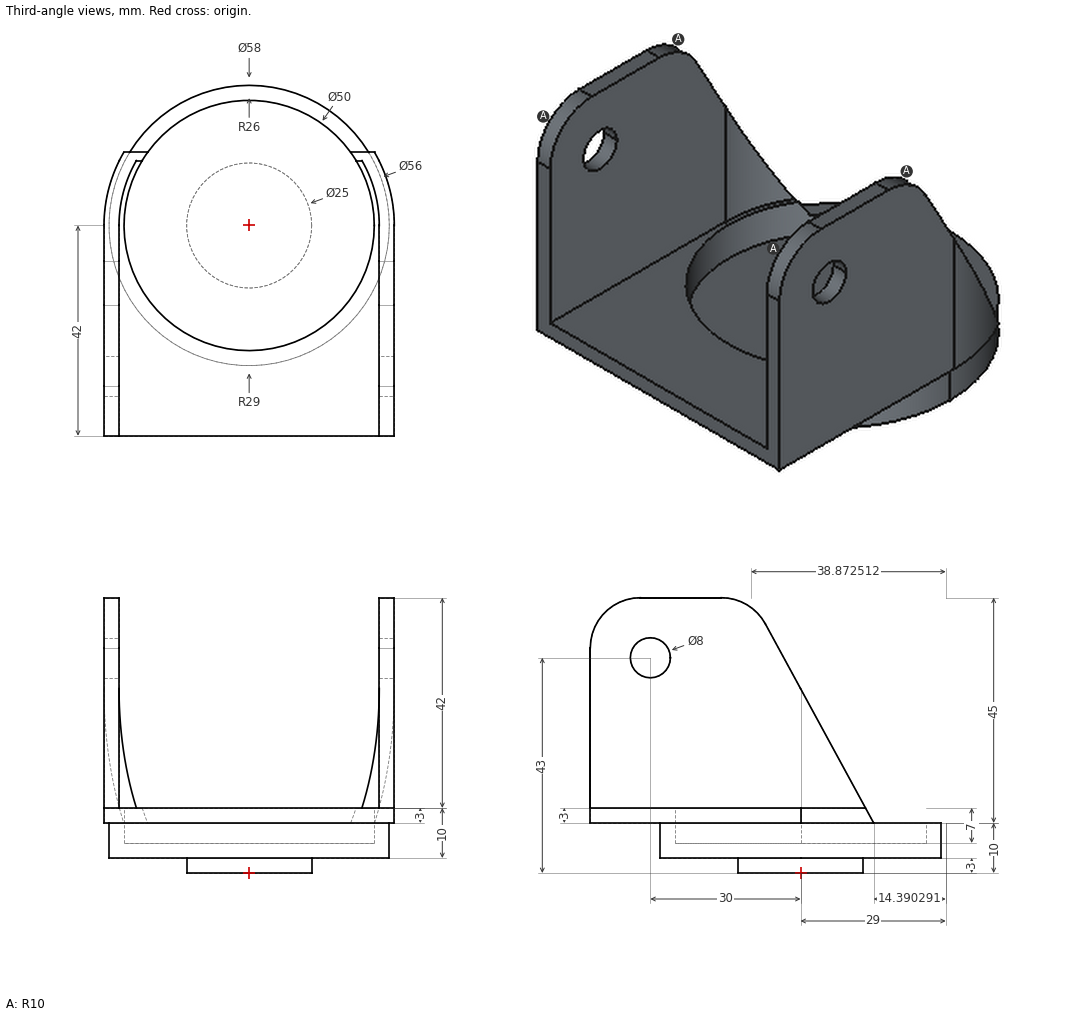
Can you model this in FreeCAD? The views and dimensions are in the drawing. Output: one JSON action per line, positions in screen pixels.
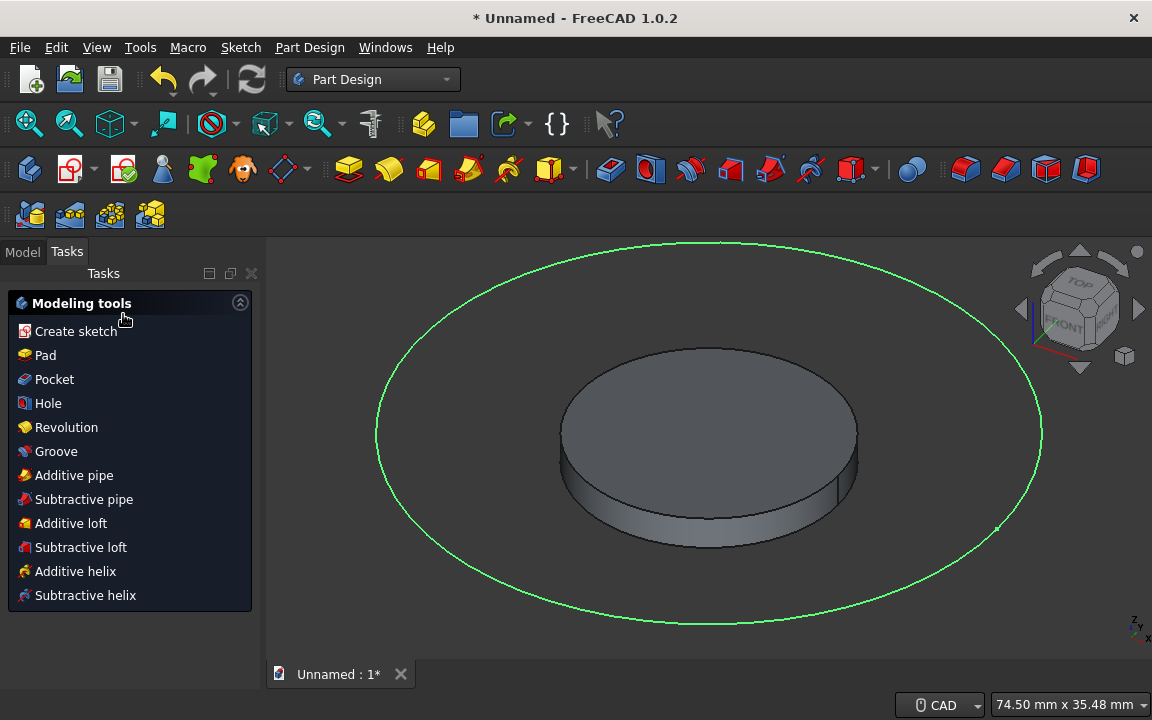
{"action": "left_click", "coordinate": [350, 170]}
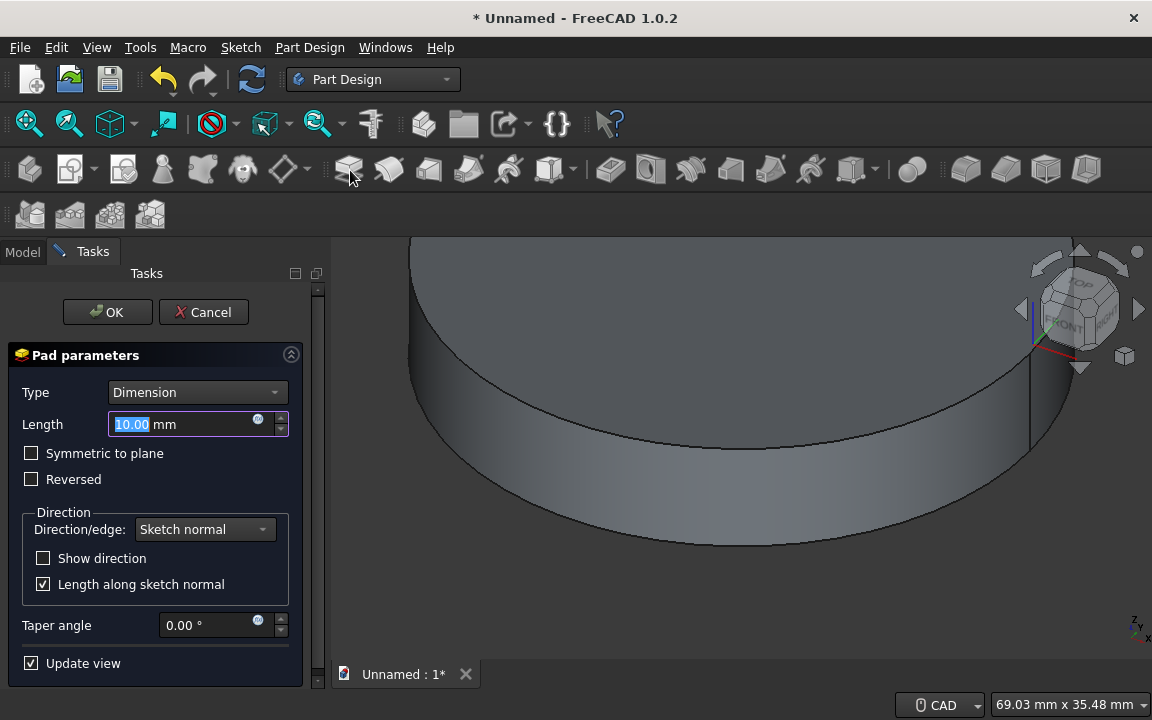
{"action": "type", "text": "10"}
{"action": "key", "text": "Tab"}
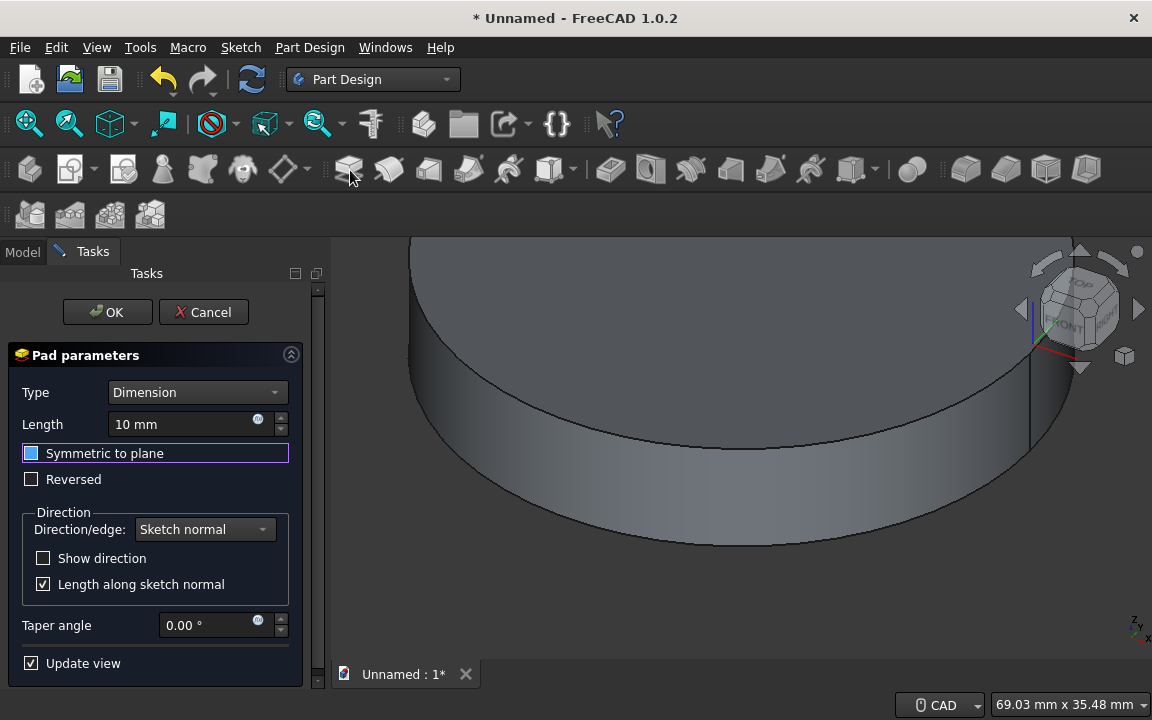
{"action": "left_click", "coordinate": [108, 312]}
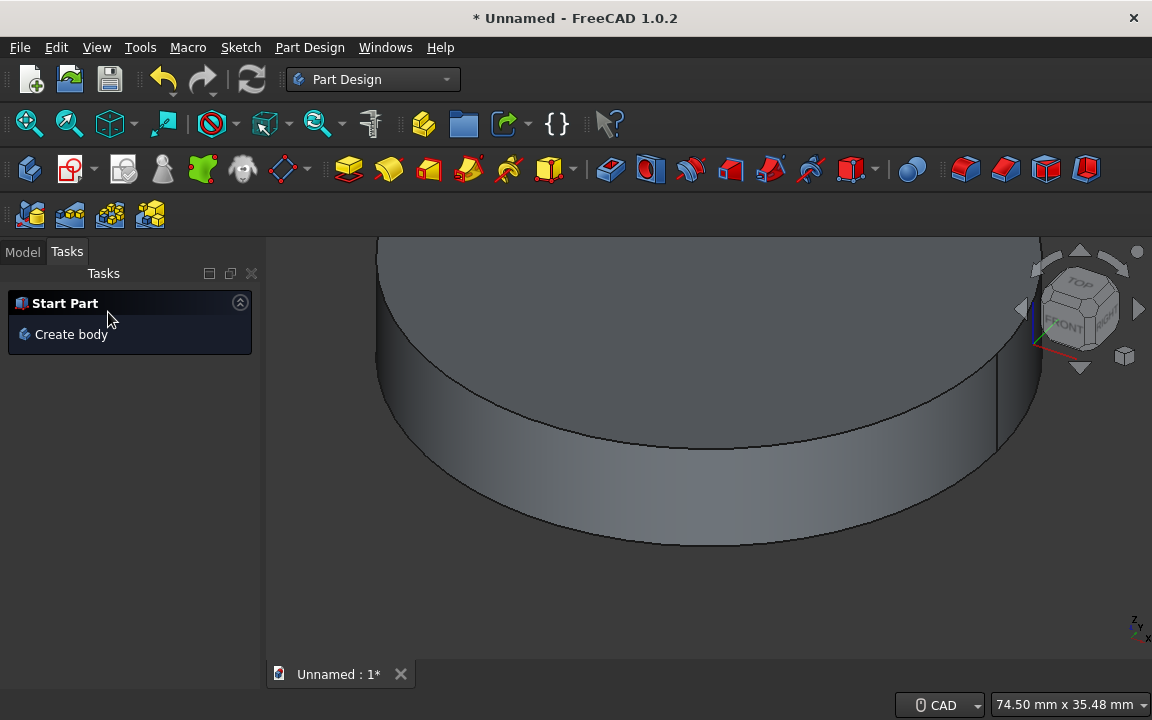
{"action": "left_click", "coordinate": [30, 124]}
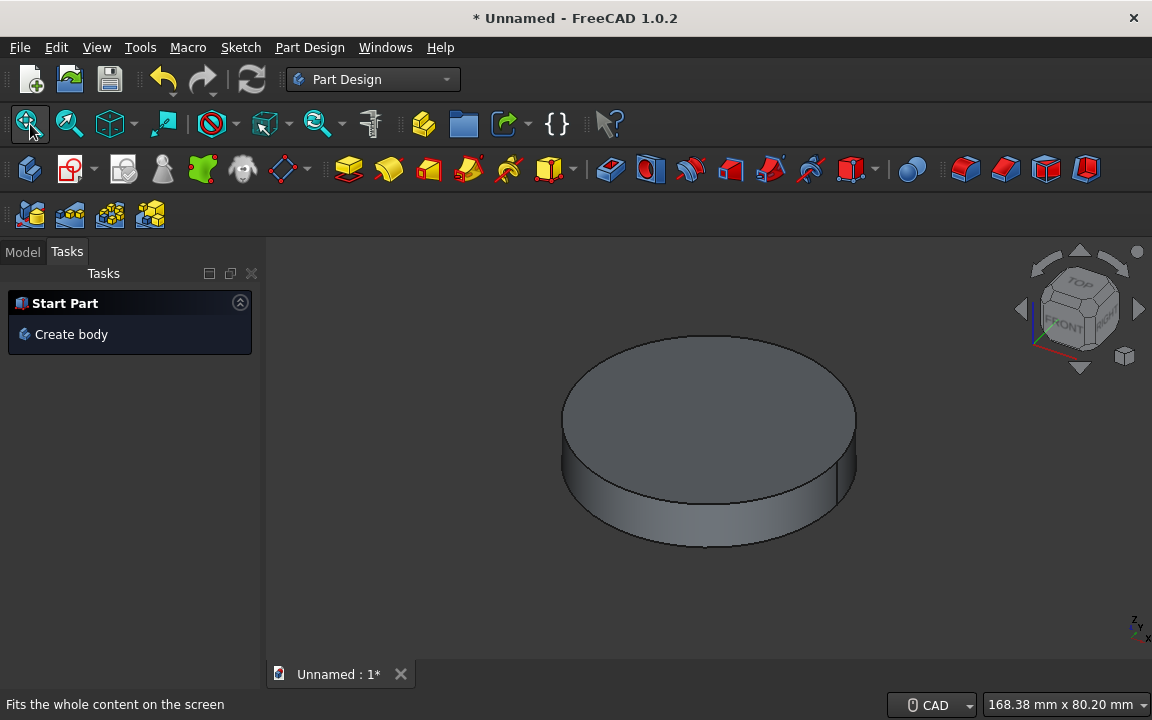
{"action": "left_click", "coordinate": [709, 419]}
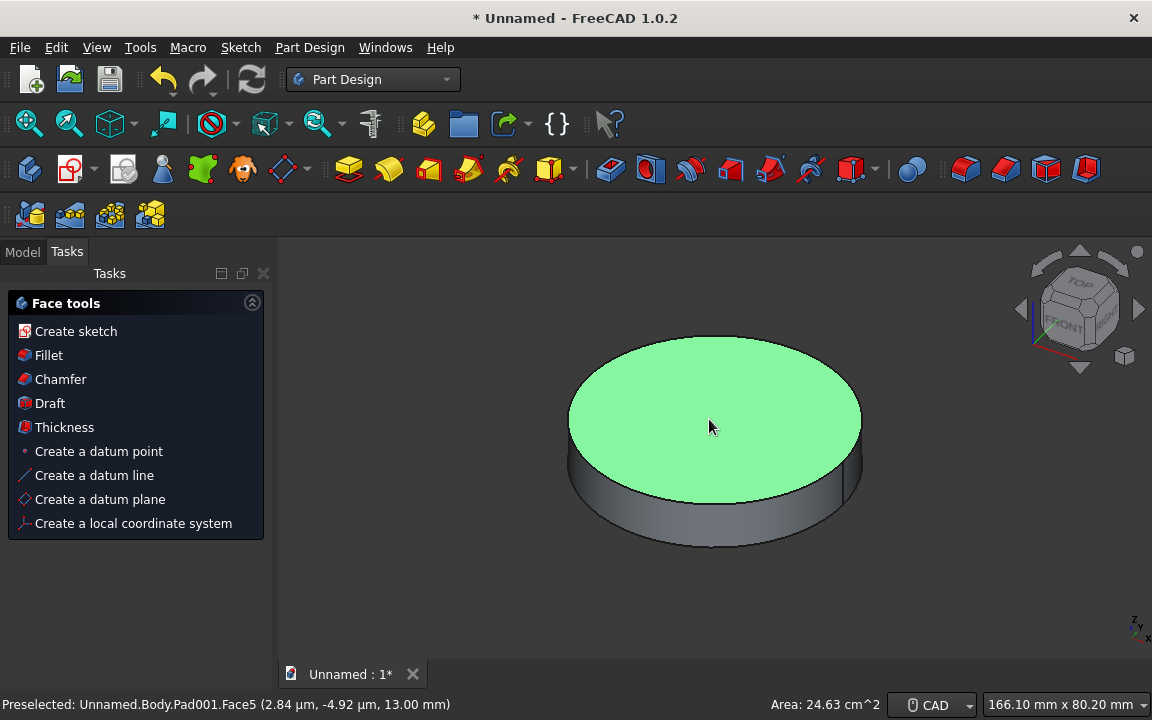
{"action": "left_click", "coordinate": [70, 170]}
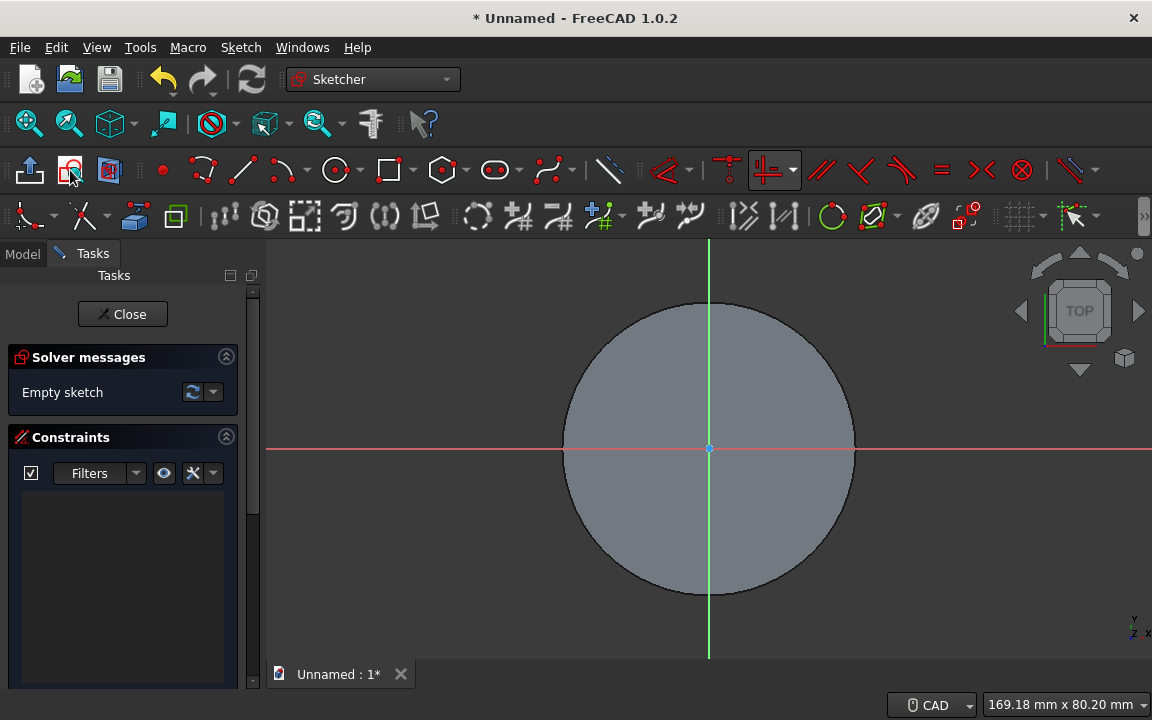
{"action": "left_click", "coordinate": [336, 170]}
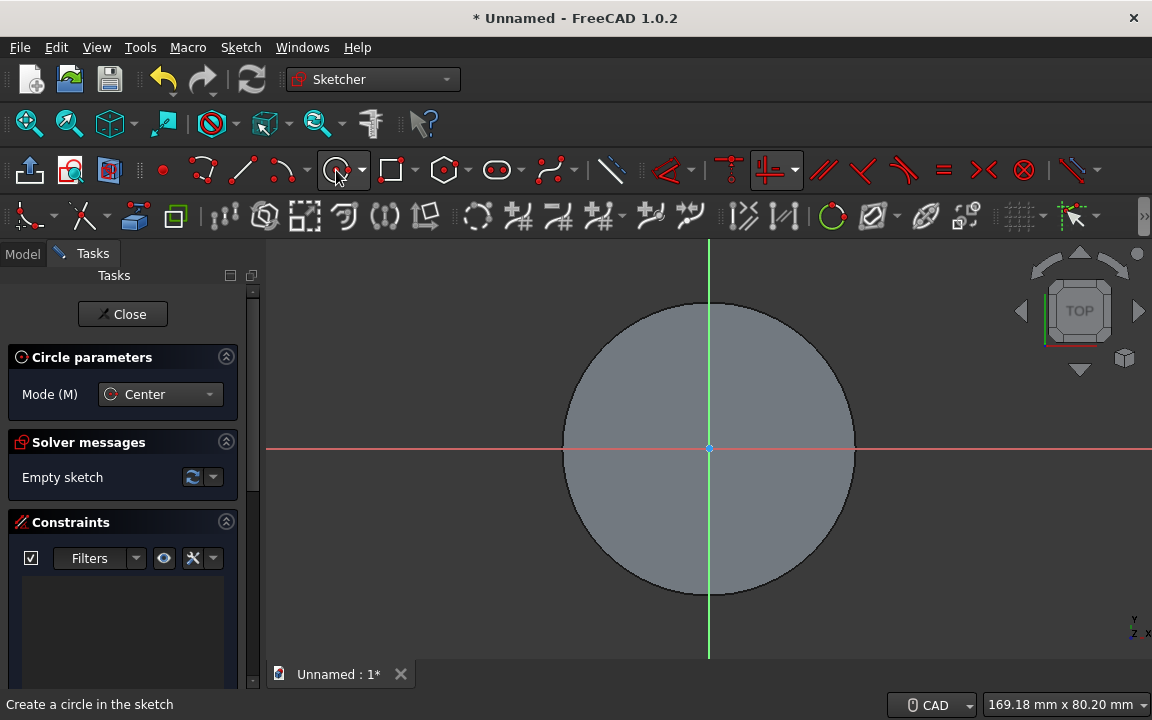
{"action": "left_click", "coordinate": [709, 449]}
{"action": "left_click", "coordinate": [802, 356]}
{"action": "key", "text": "Escape"}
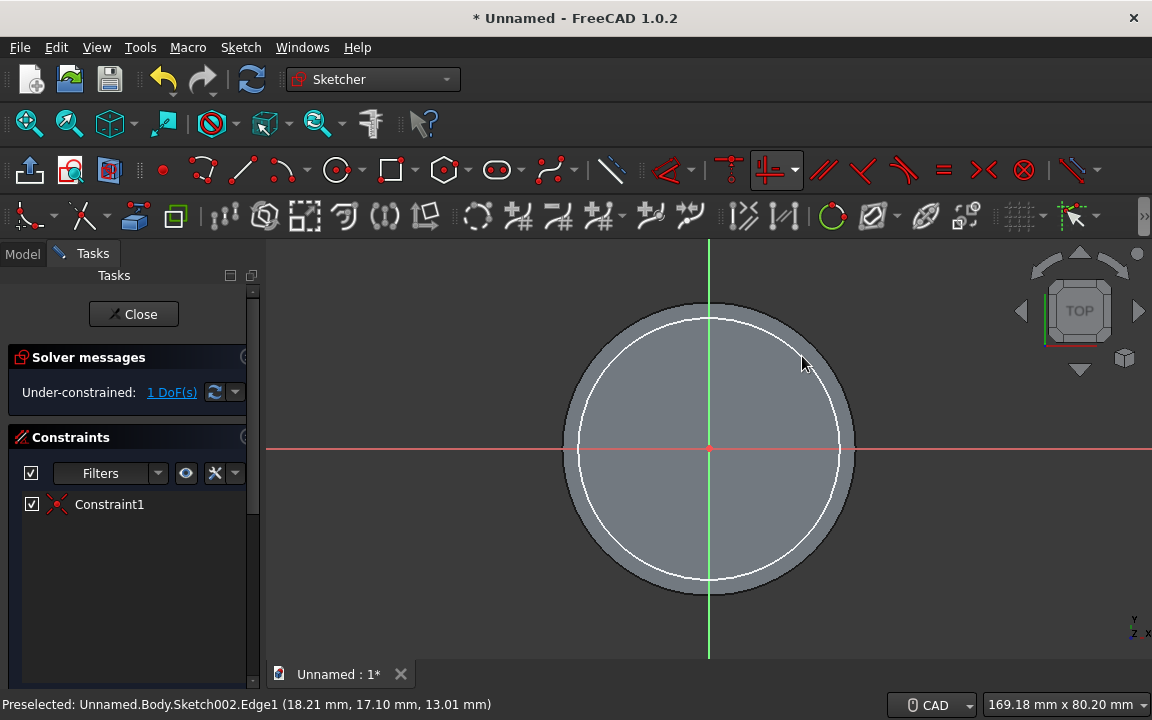
{"action": "left_click", "coordinate": [666, 170]}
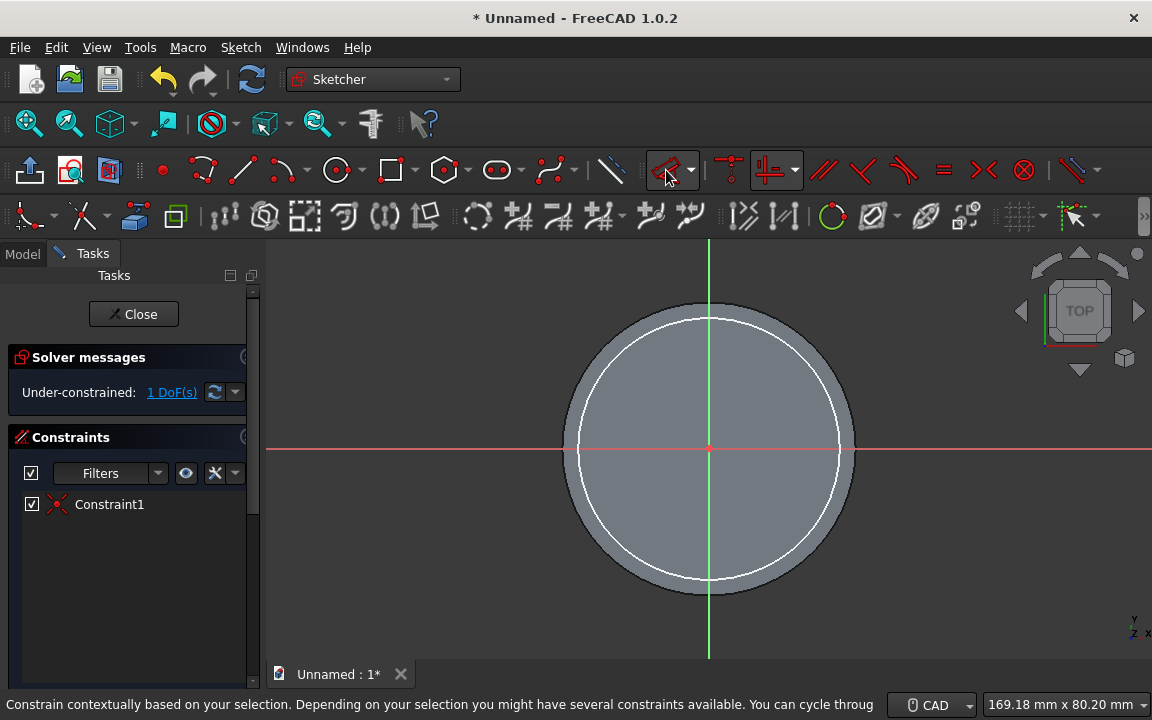
{"action": "left_click", "coordinate": [801, 356]}
{"action": "left_click", "coordinate": [824, 333]}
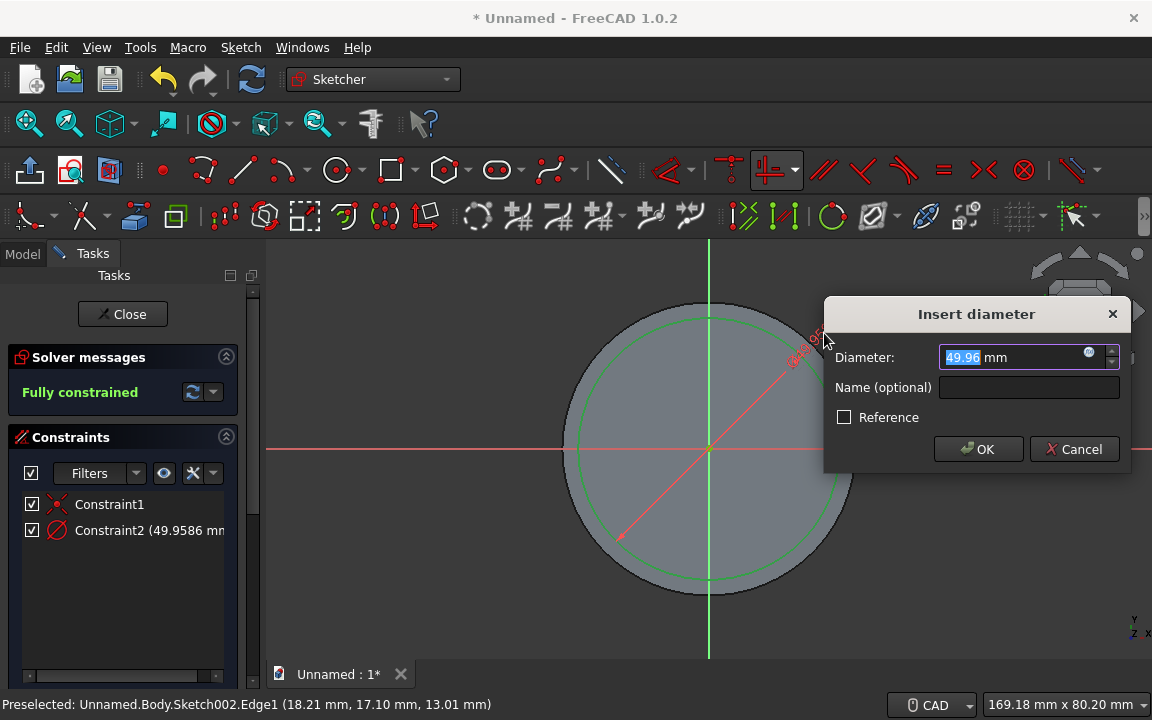
{"action": "type", "text": "50"}
{"action": "key", "text": "Return"}
{"action": "key", "text": "Escape"}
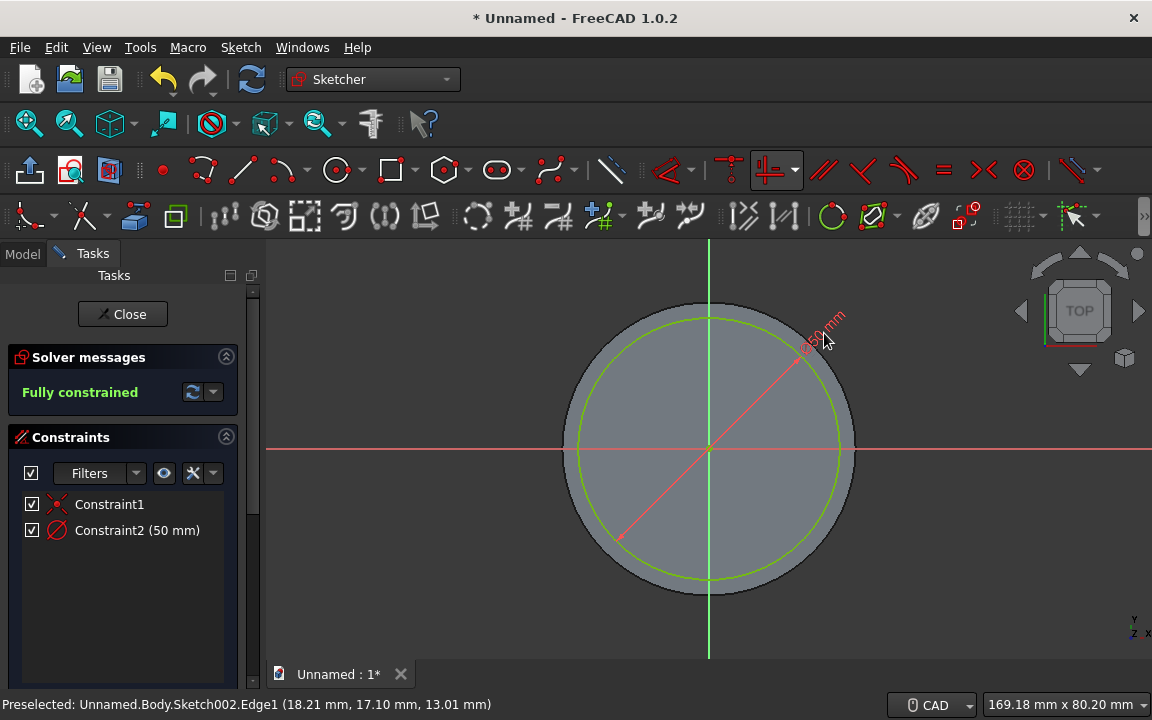
{"action": "left_click", "coordinate": [123, 314]}